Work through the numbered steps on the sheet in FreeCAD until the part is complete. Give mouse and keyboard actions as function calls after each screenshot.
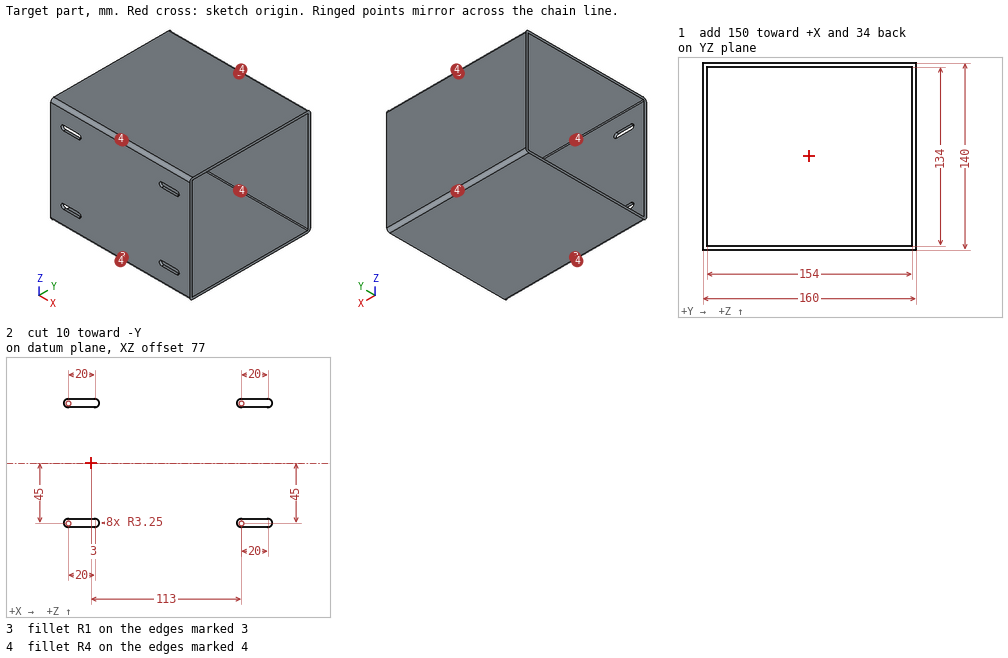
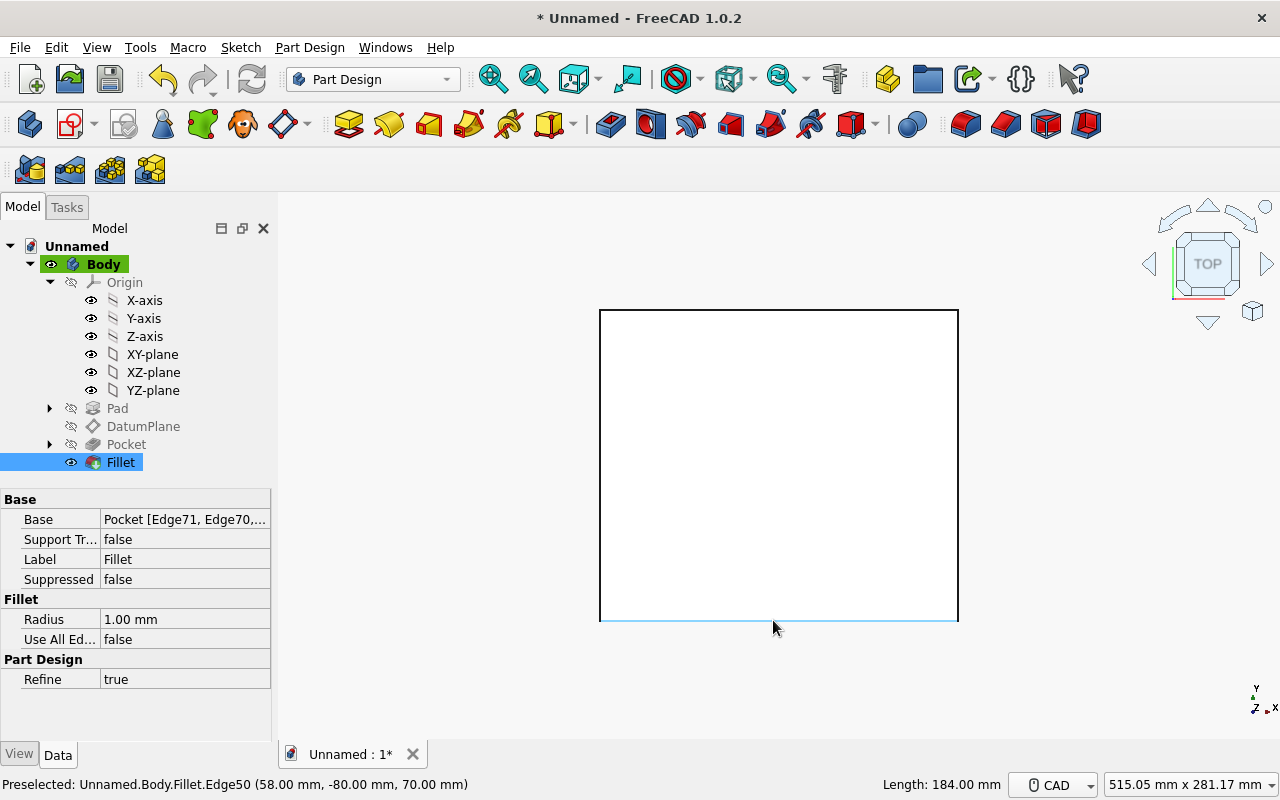
click(779, 309, ctrl)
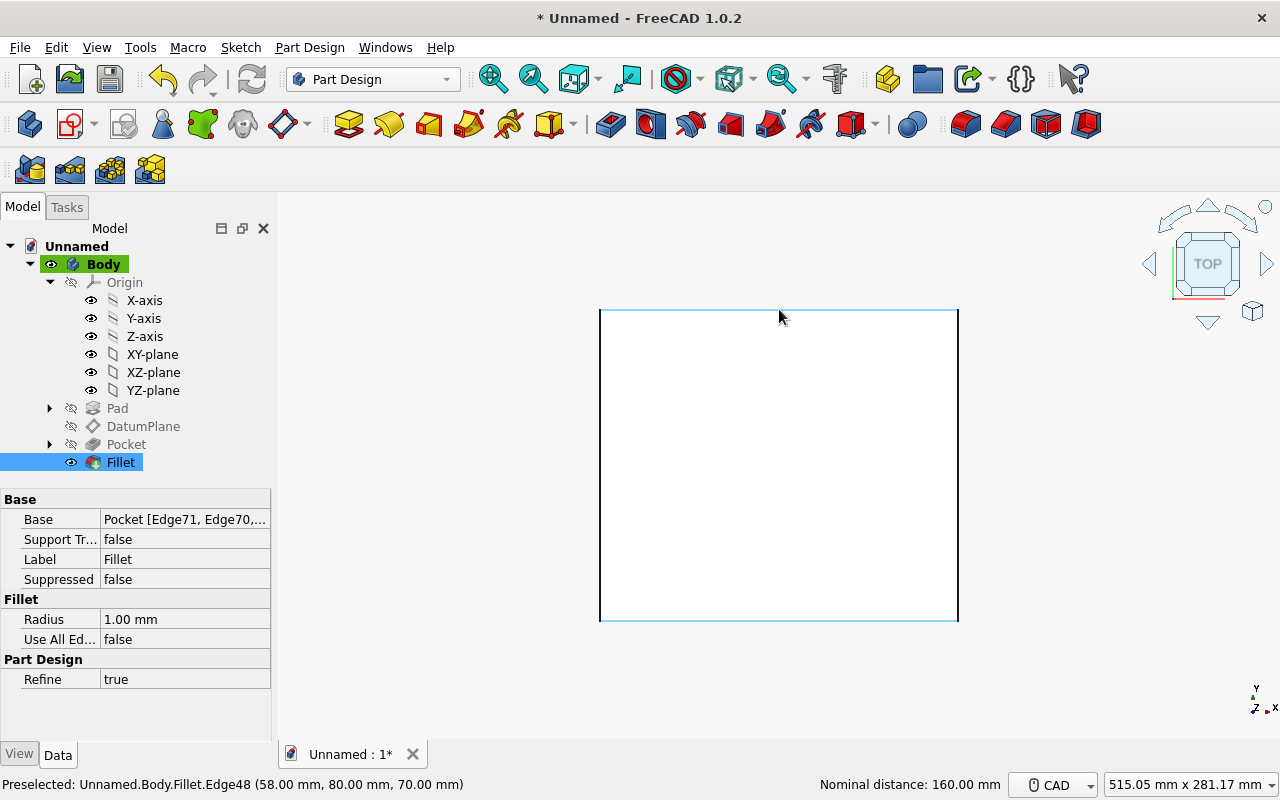
key(0)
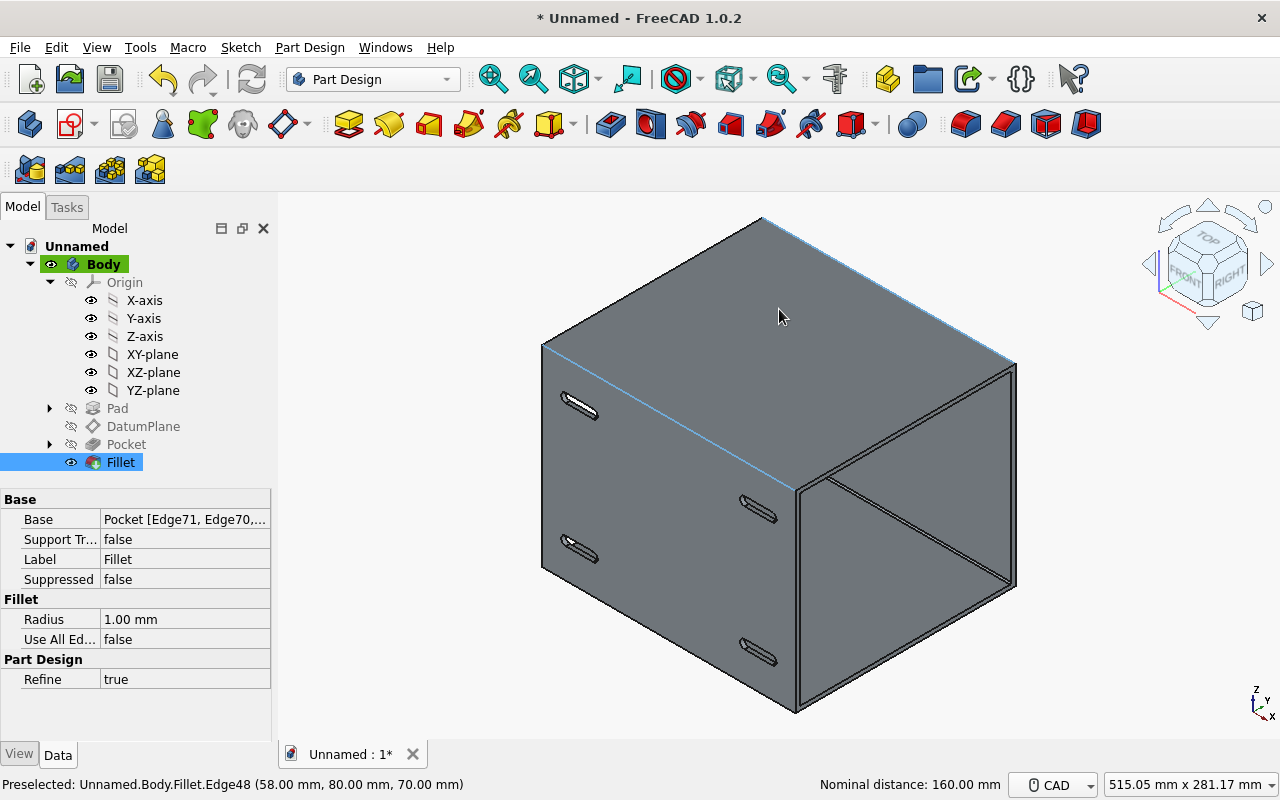
key(2)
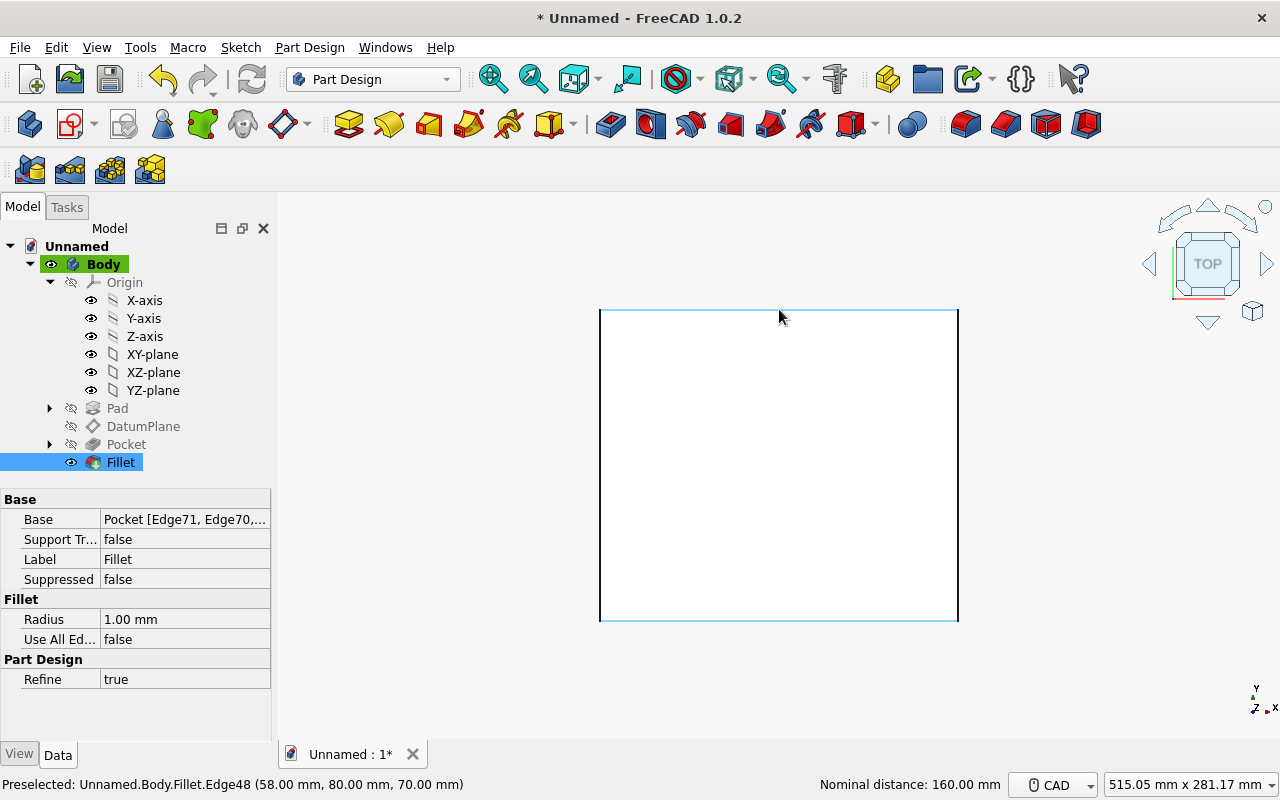
key(1)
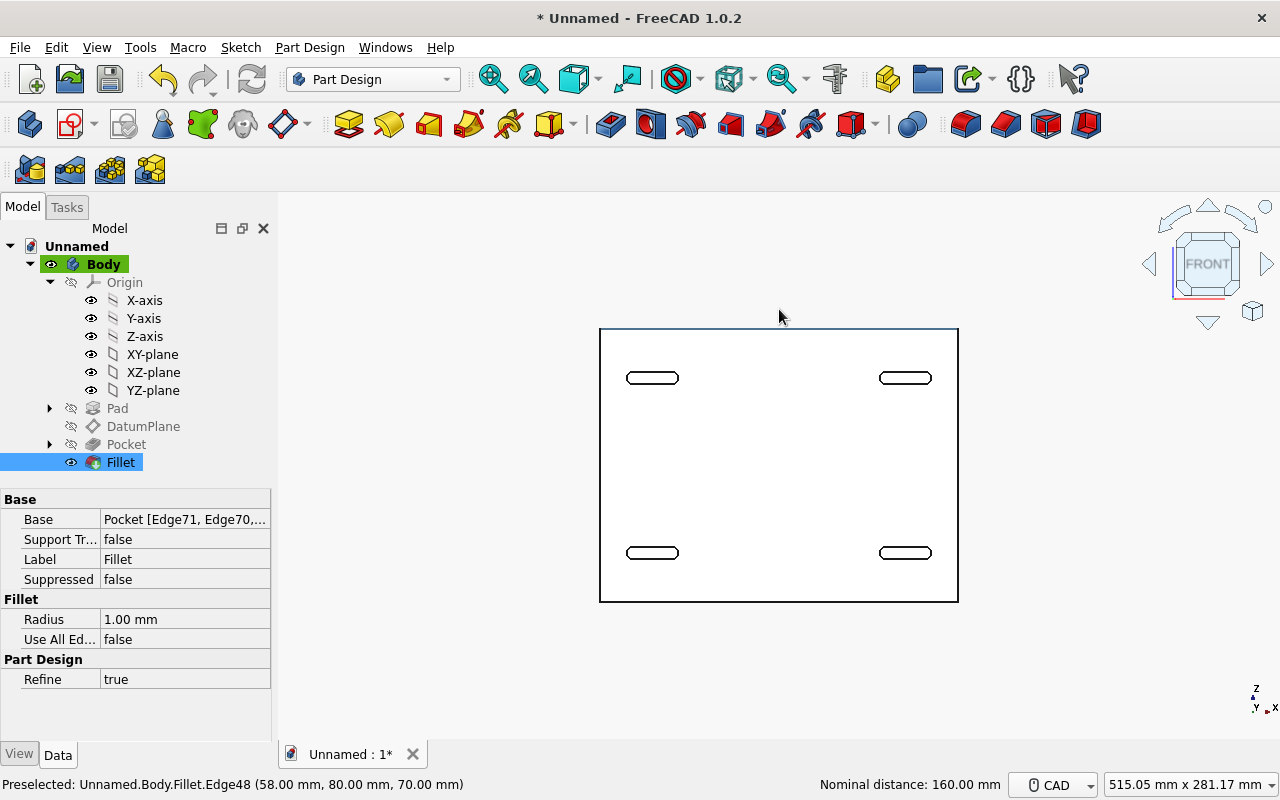
click(779, 601, ctrl)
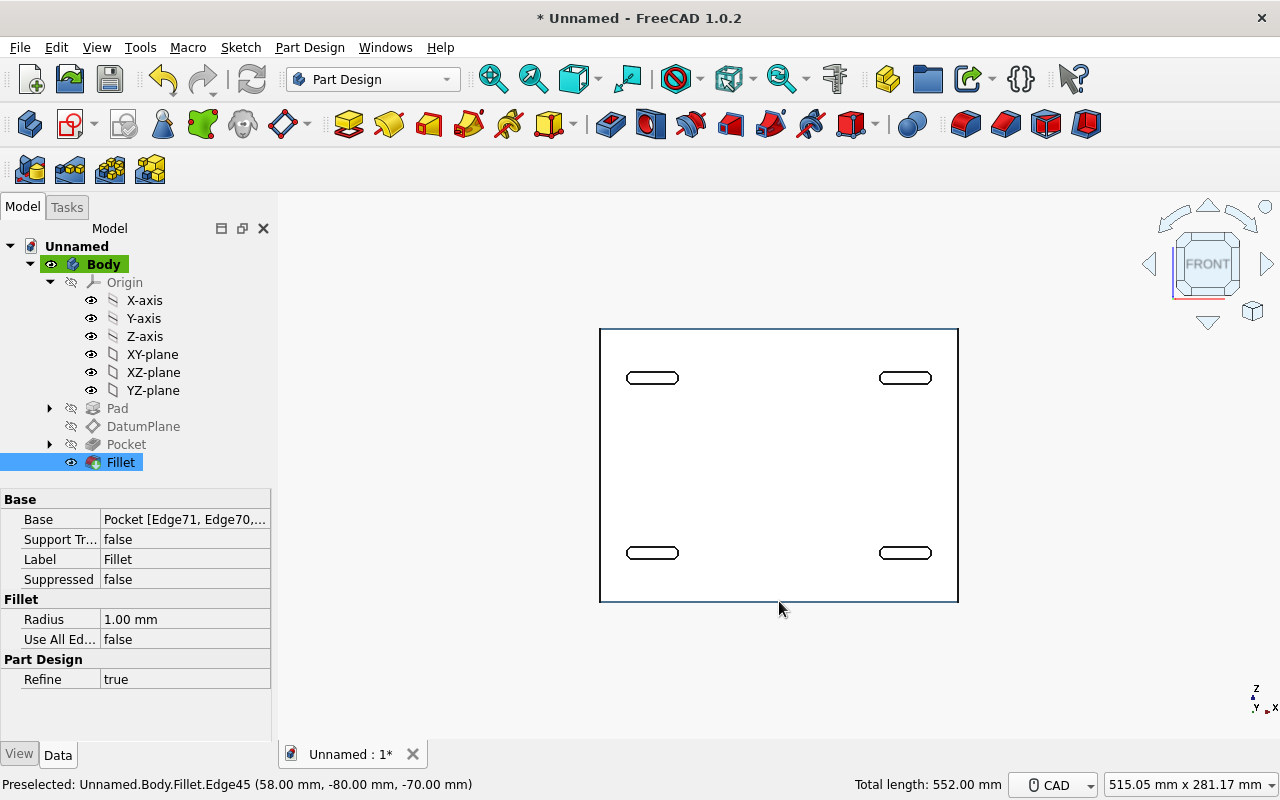
key(3)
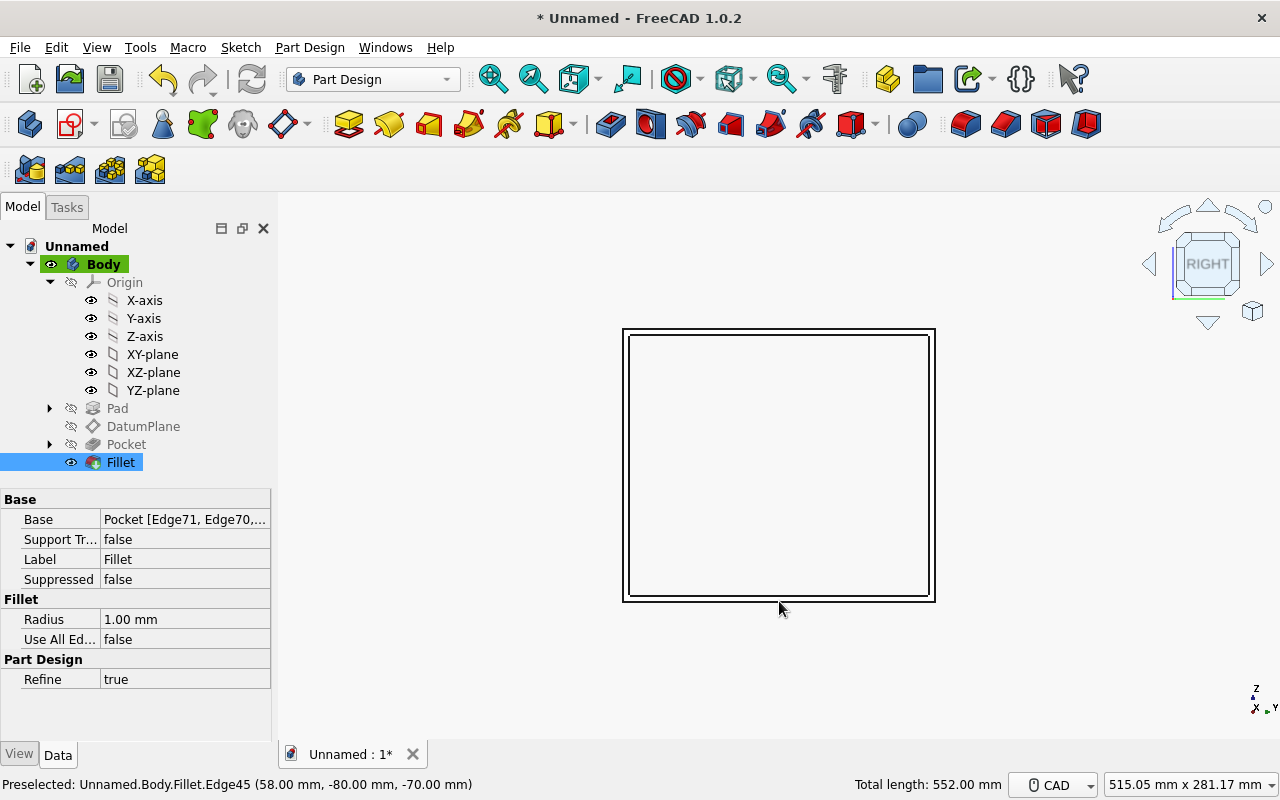
key(5)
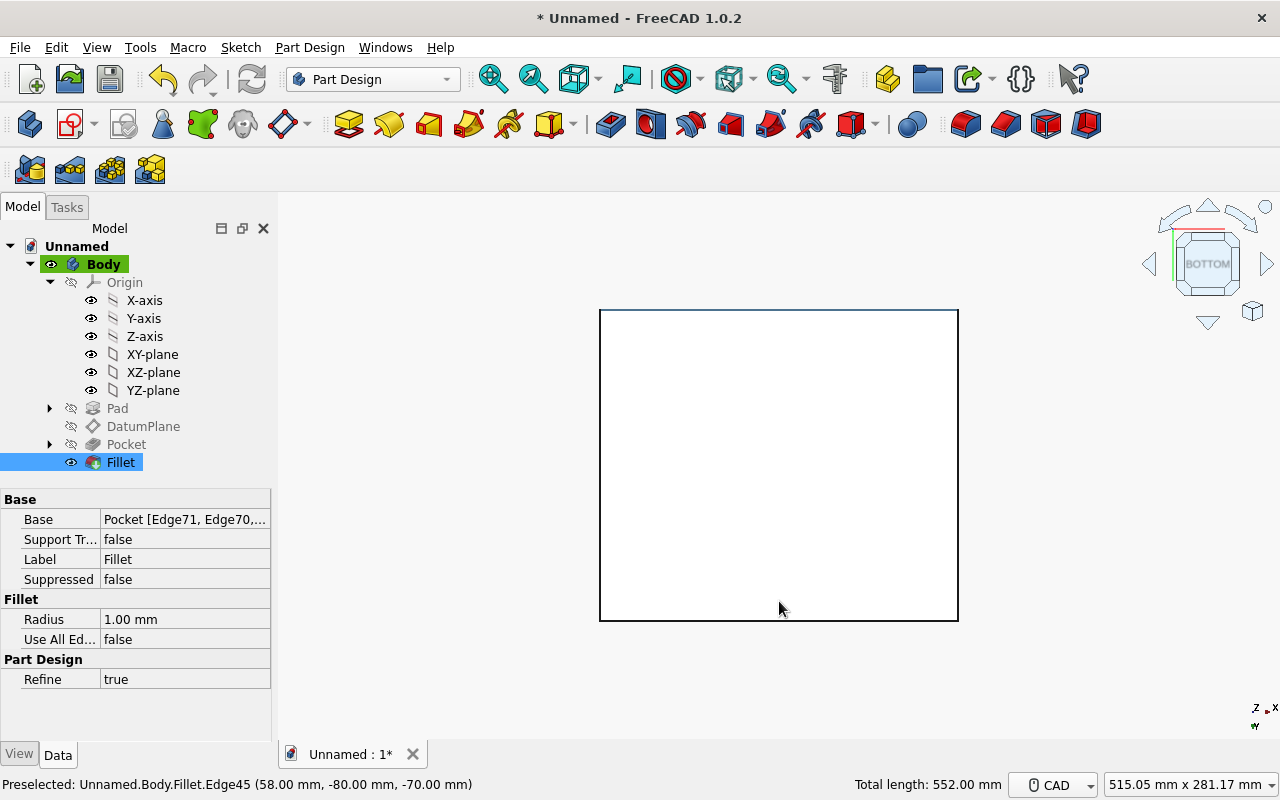
click(779, 620, ctrl)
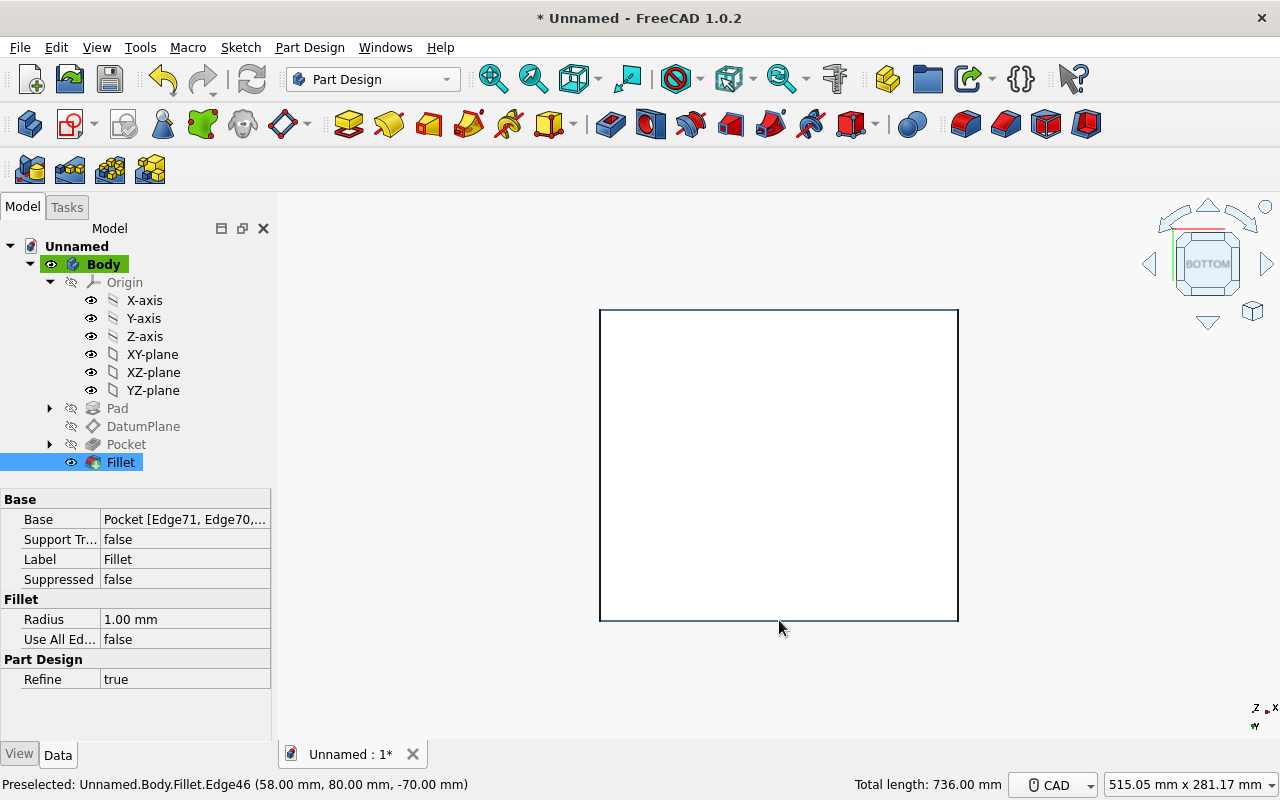
click(966, 124)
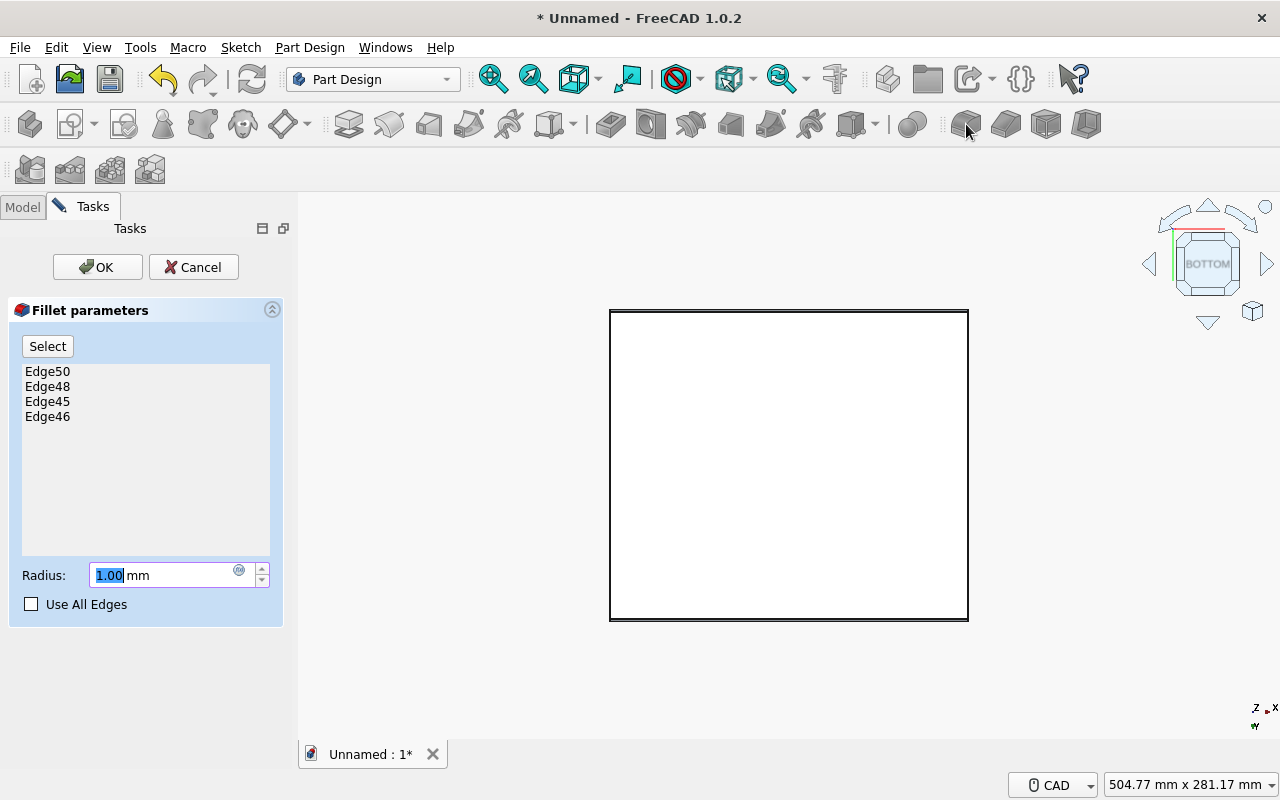
text(4)
key(Tab)